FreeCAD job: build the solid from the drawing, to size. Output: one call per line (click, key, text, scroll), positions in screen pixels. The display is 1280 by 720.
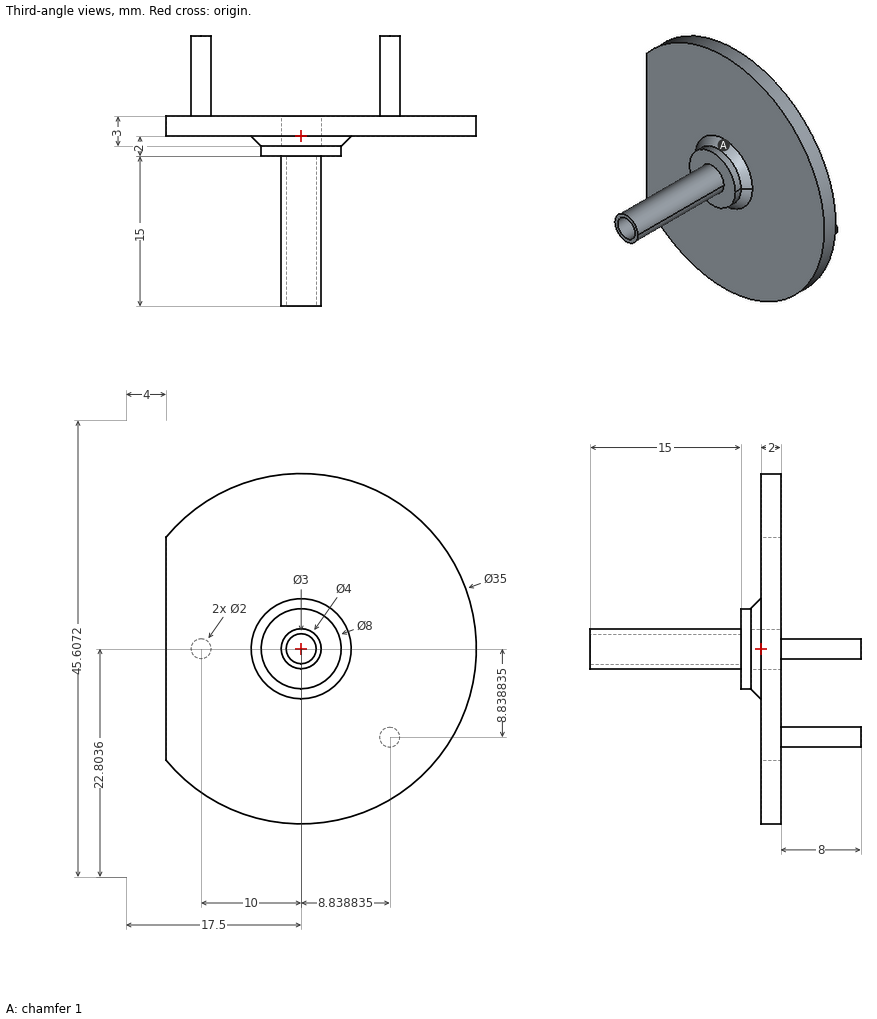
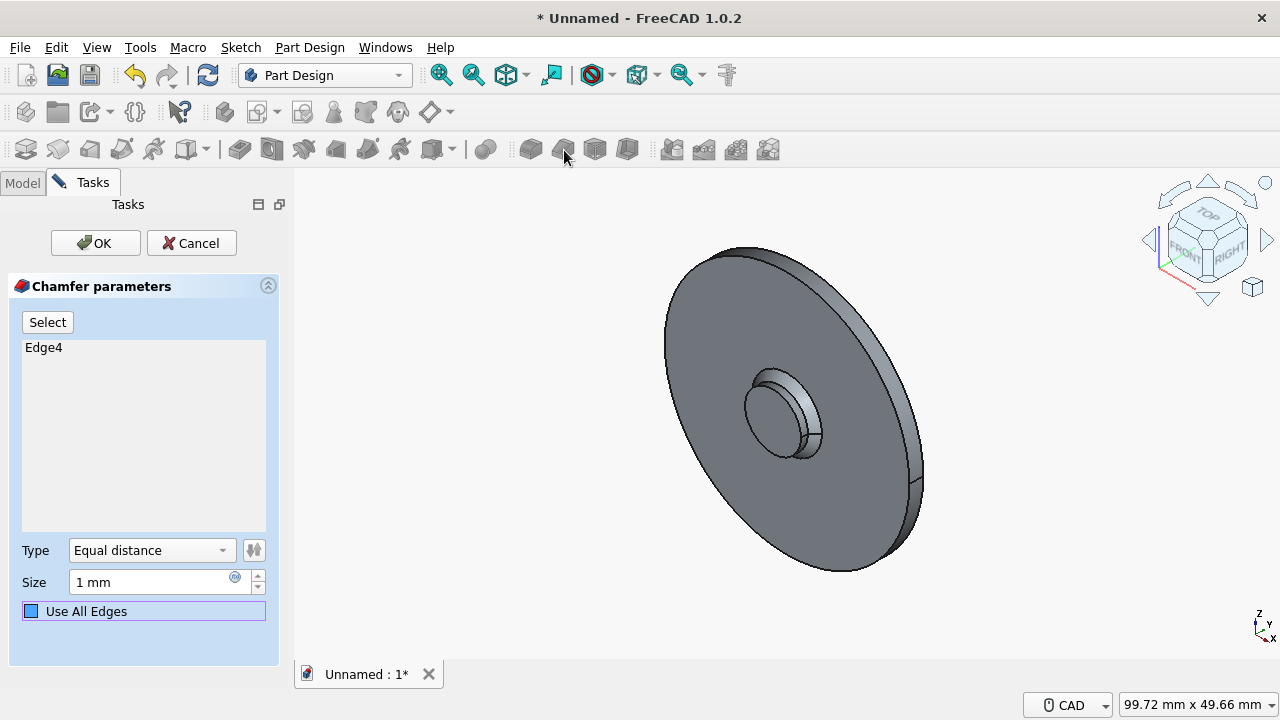
click(96, 243)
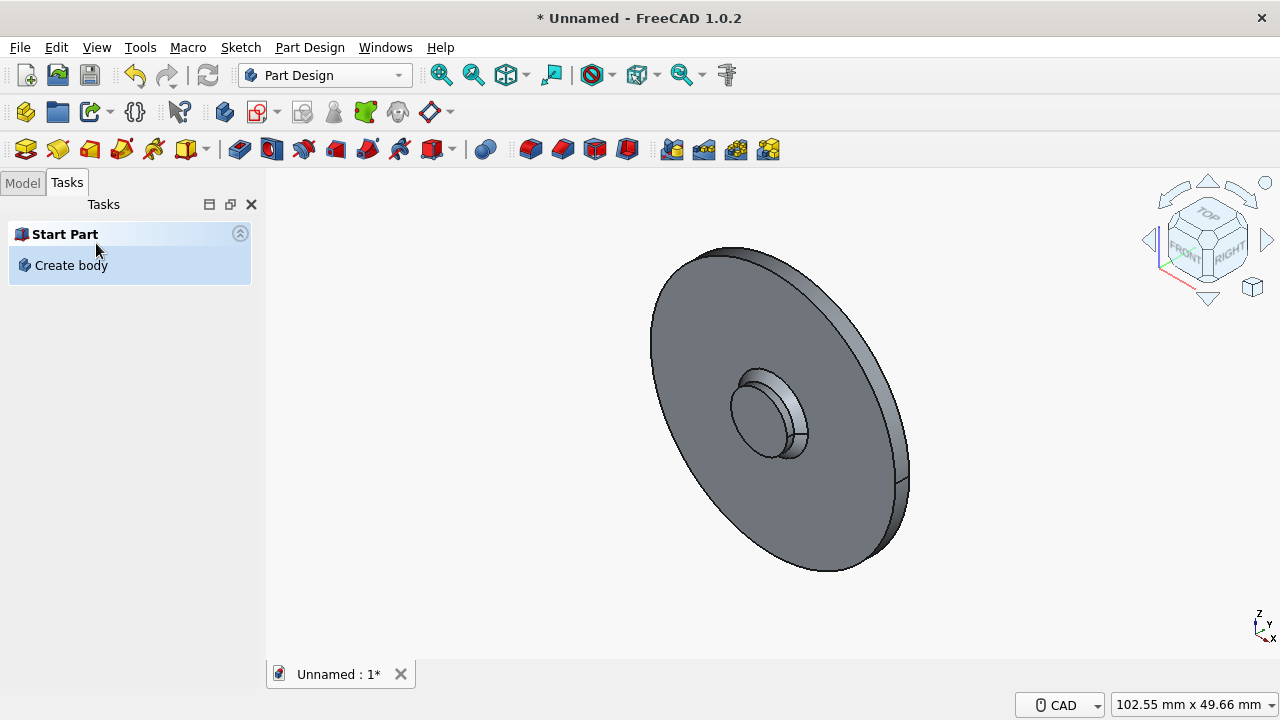
click(759, 421)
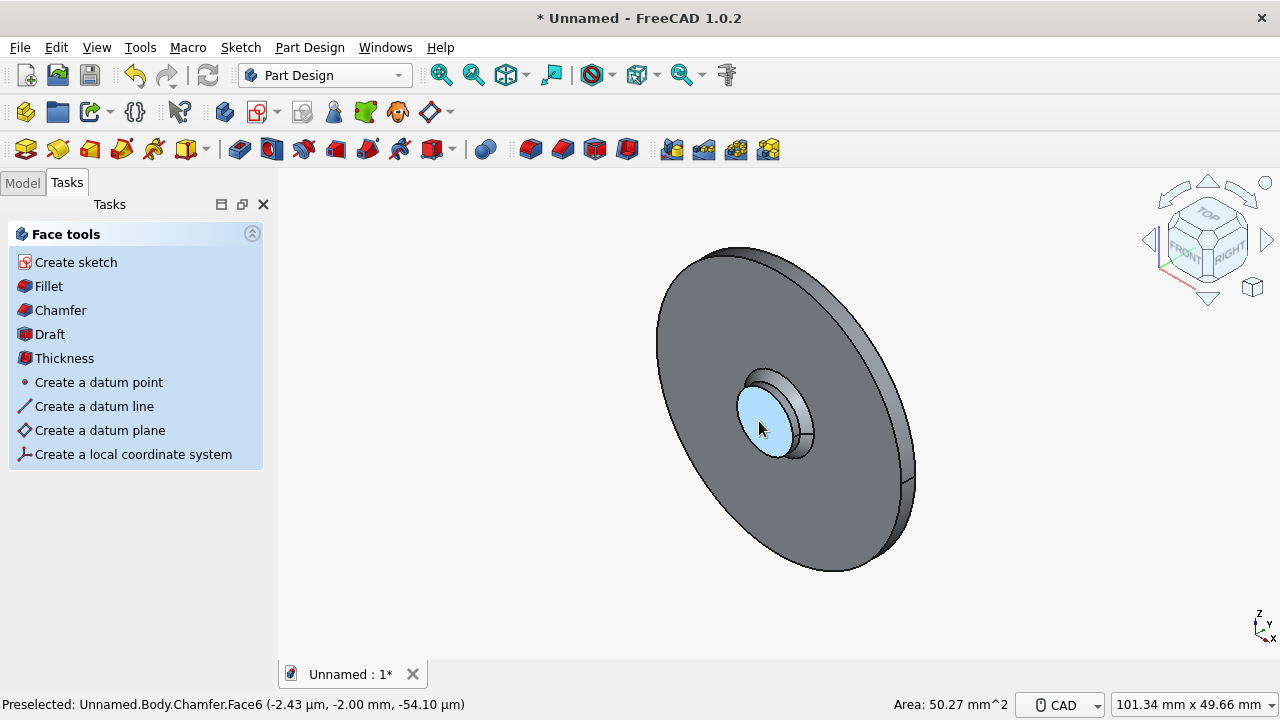
click(258, 112)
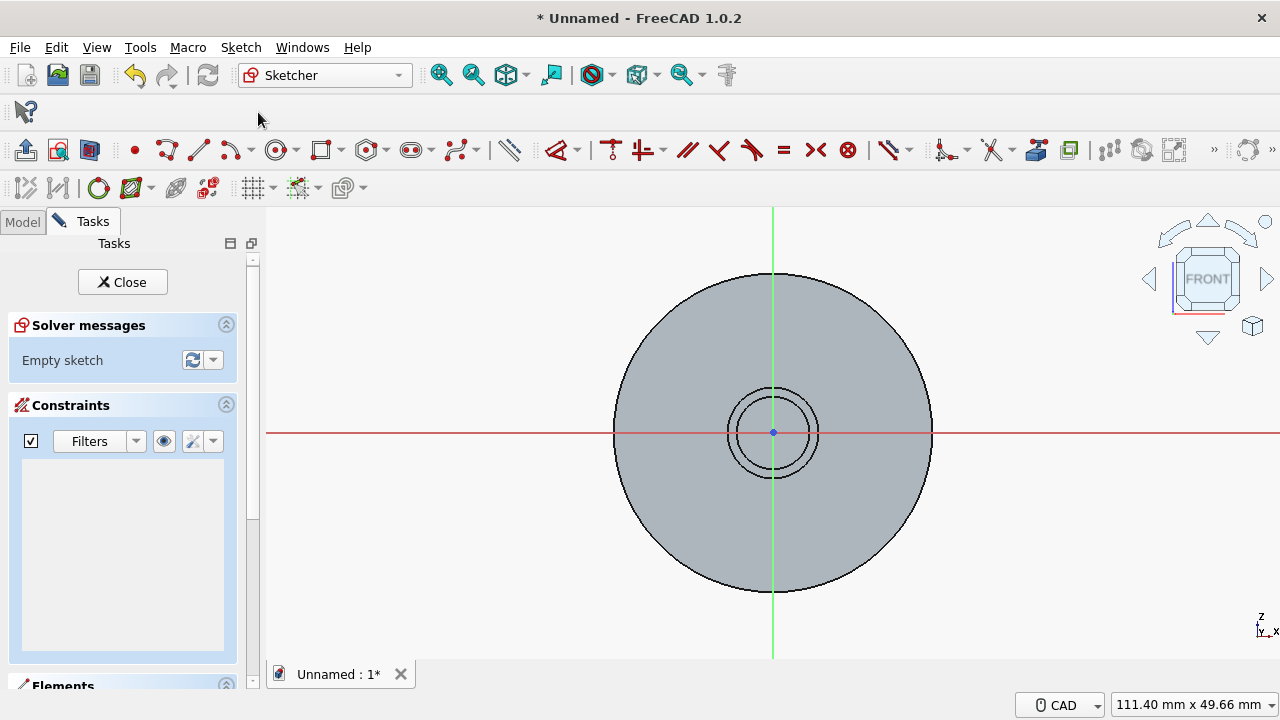
scroll(784, 433, up, 10)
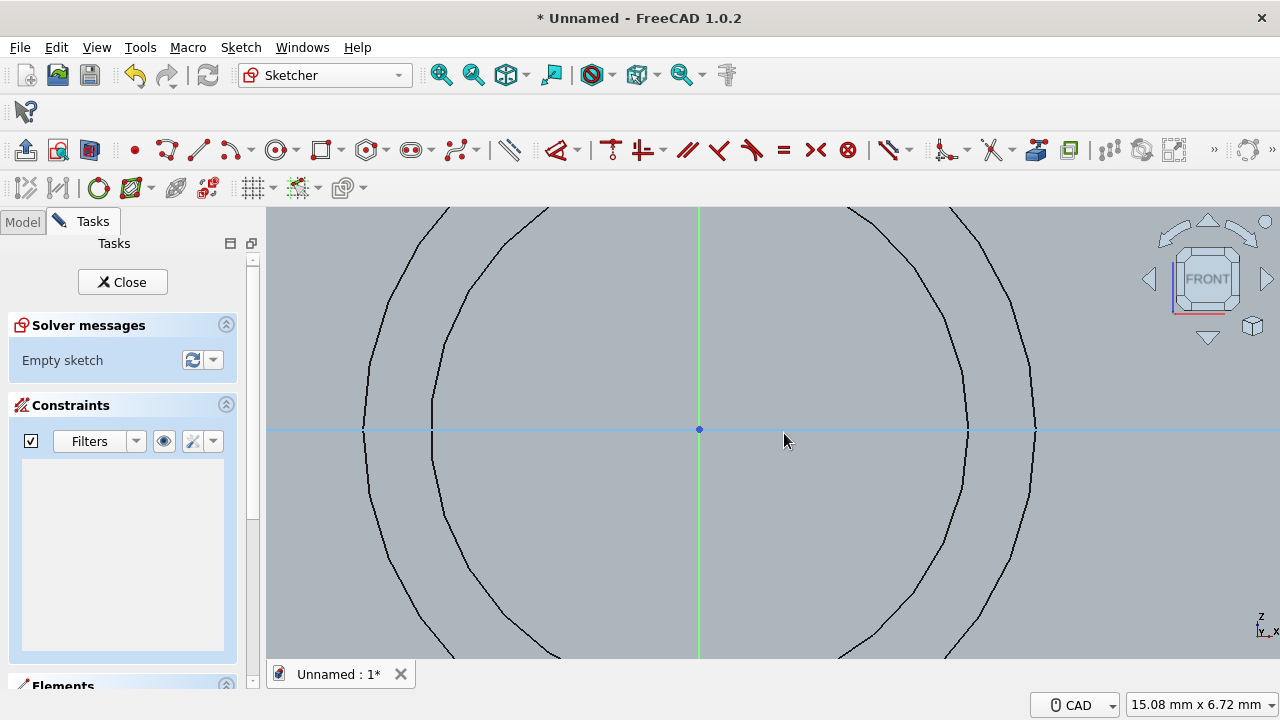
click(276, 150)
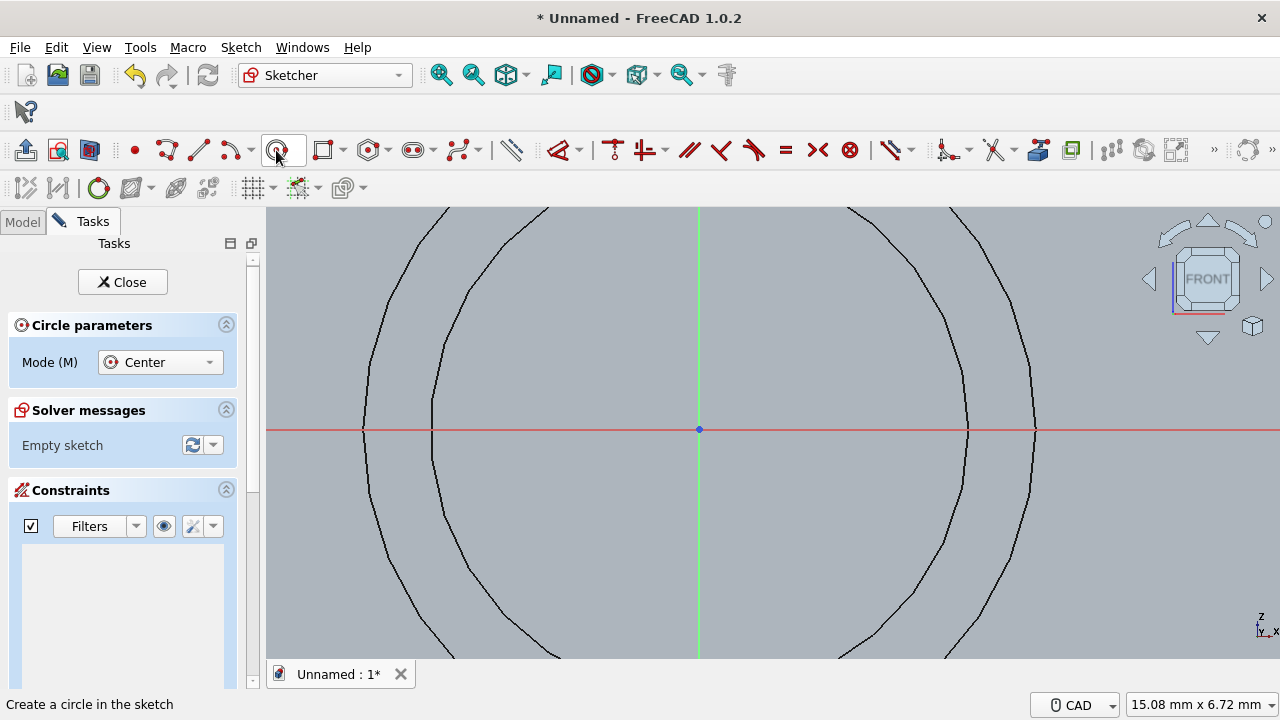
click(699, 430)
click(795, 335)
key(Escape)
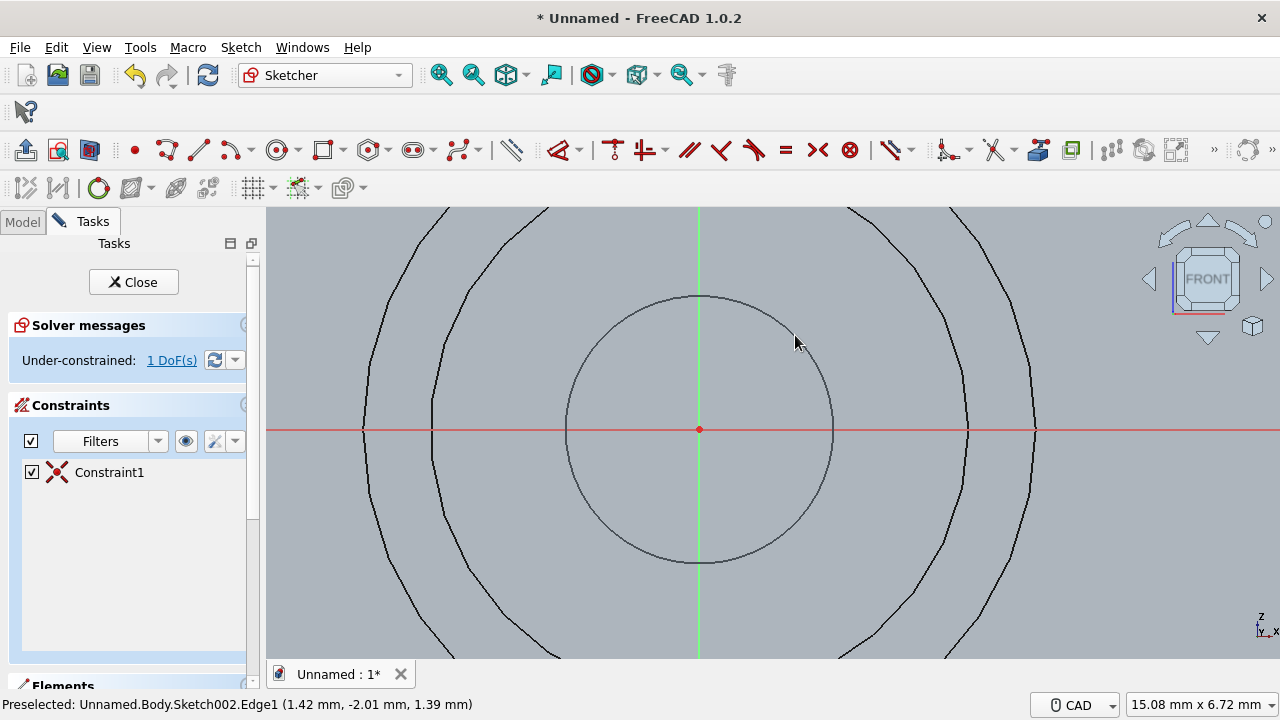
click(558, 150)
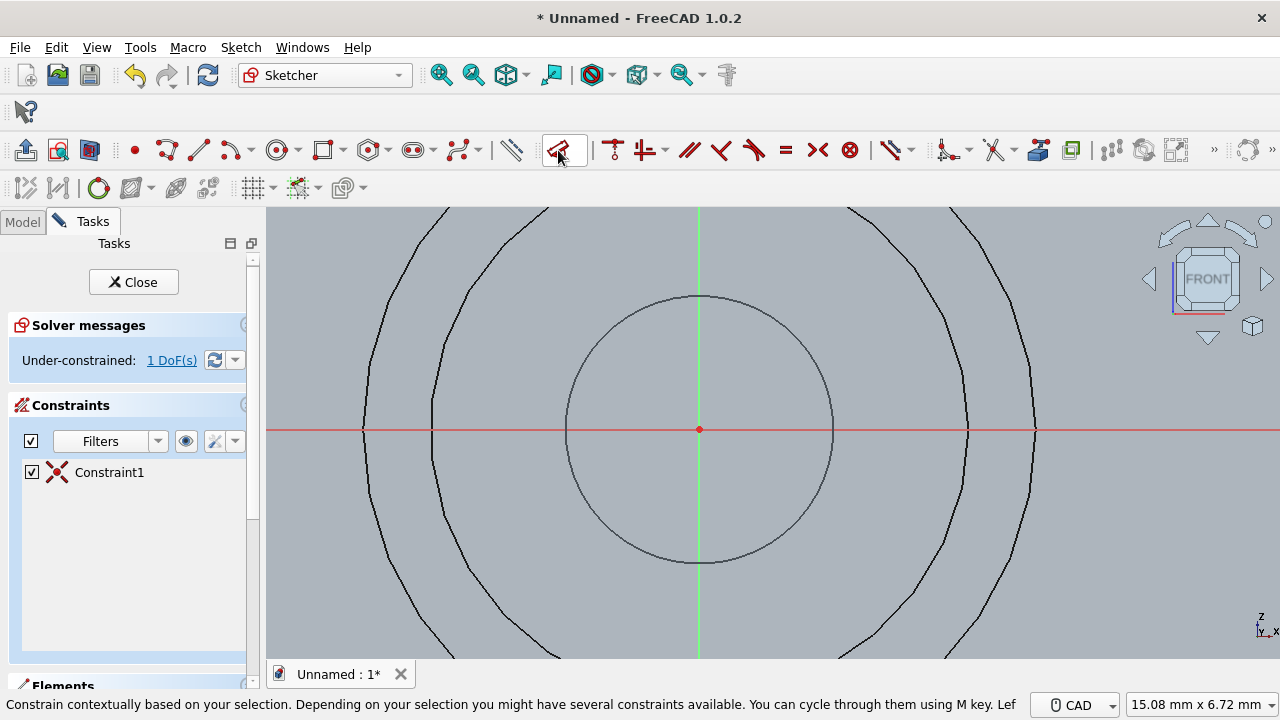
click(794, 335)
click(817, 312)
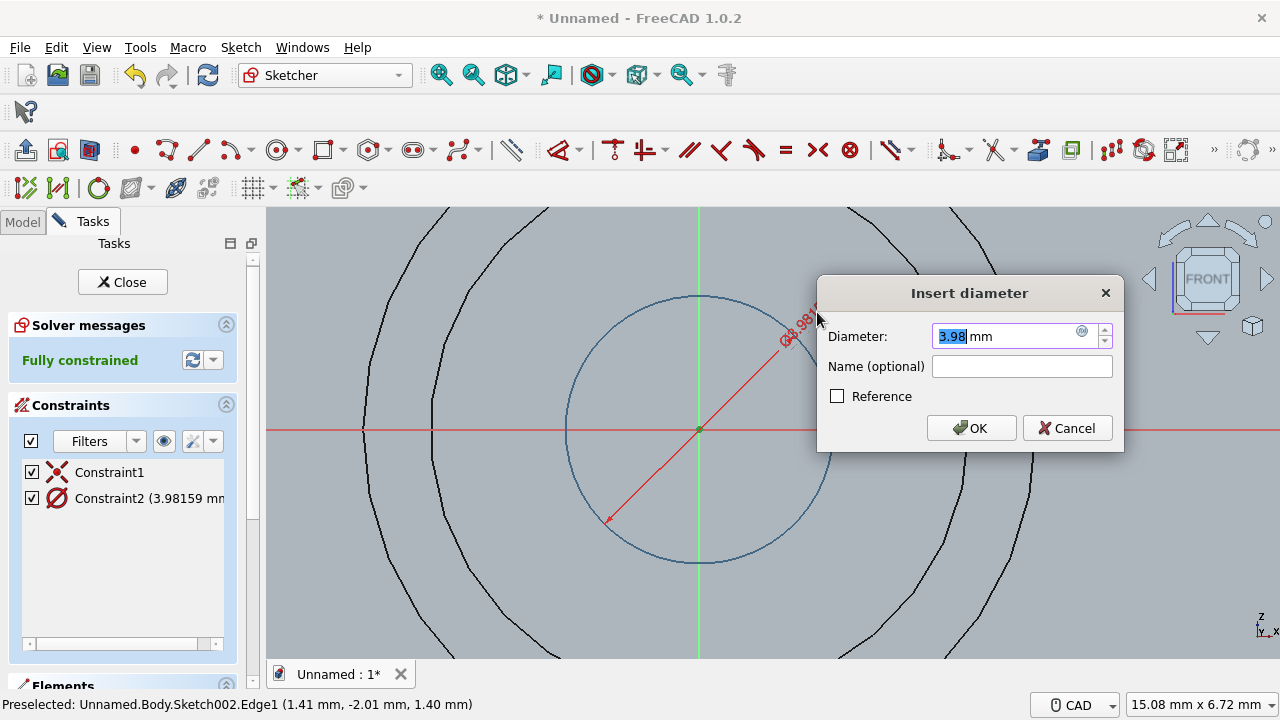
text(4)
key(Return)
key(Escape)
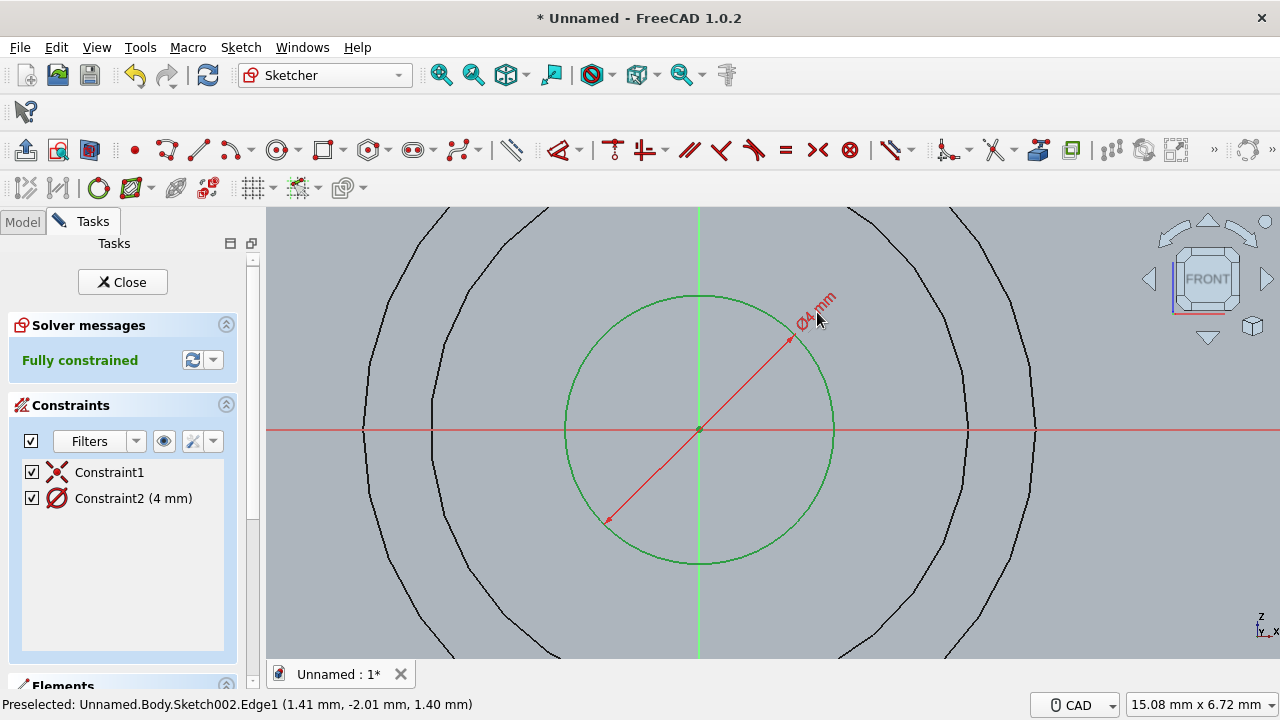
click(123, 282)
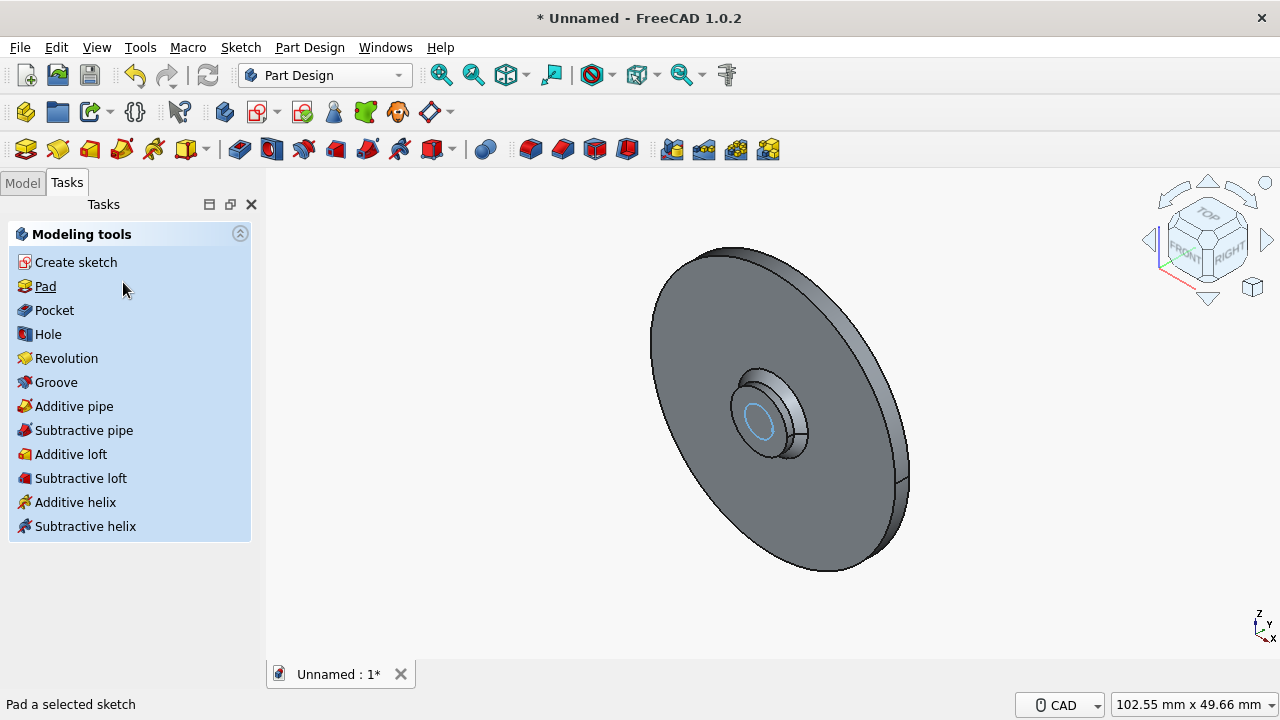
click(26, 150)